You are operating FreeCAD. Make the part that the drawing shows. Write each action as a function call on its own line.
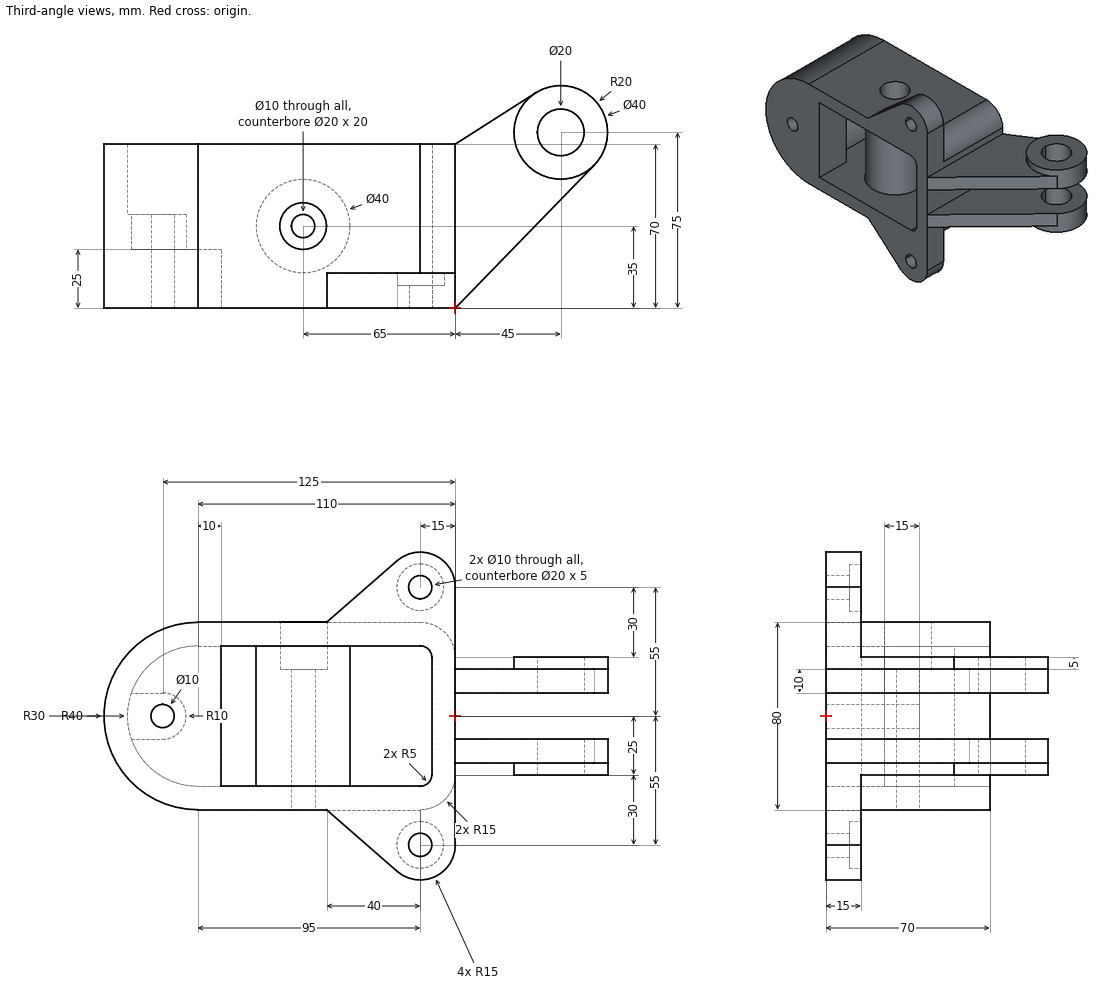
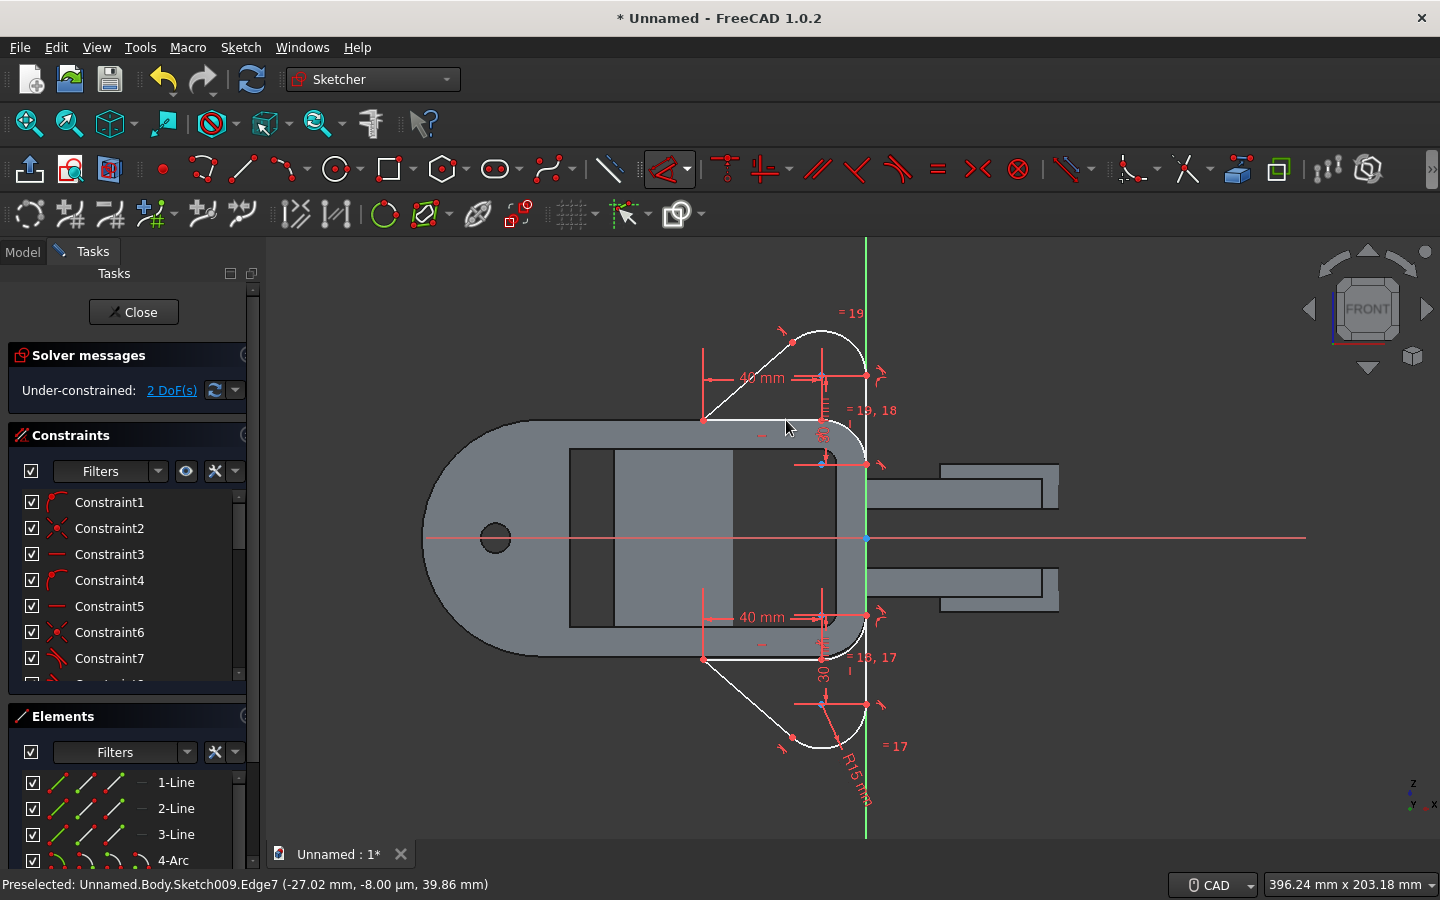
click(866, 615)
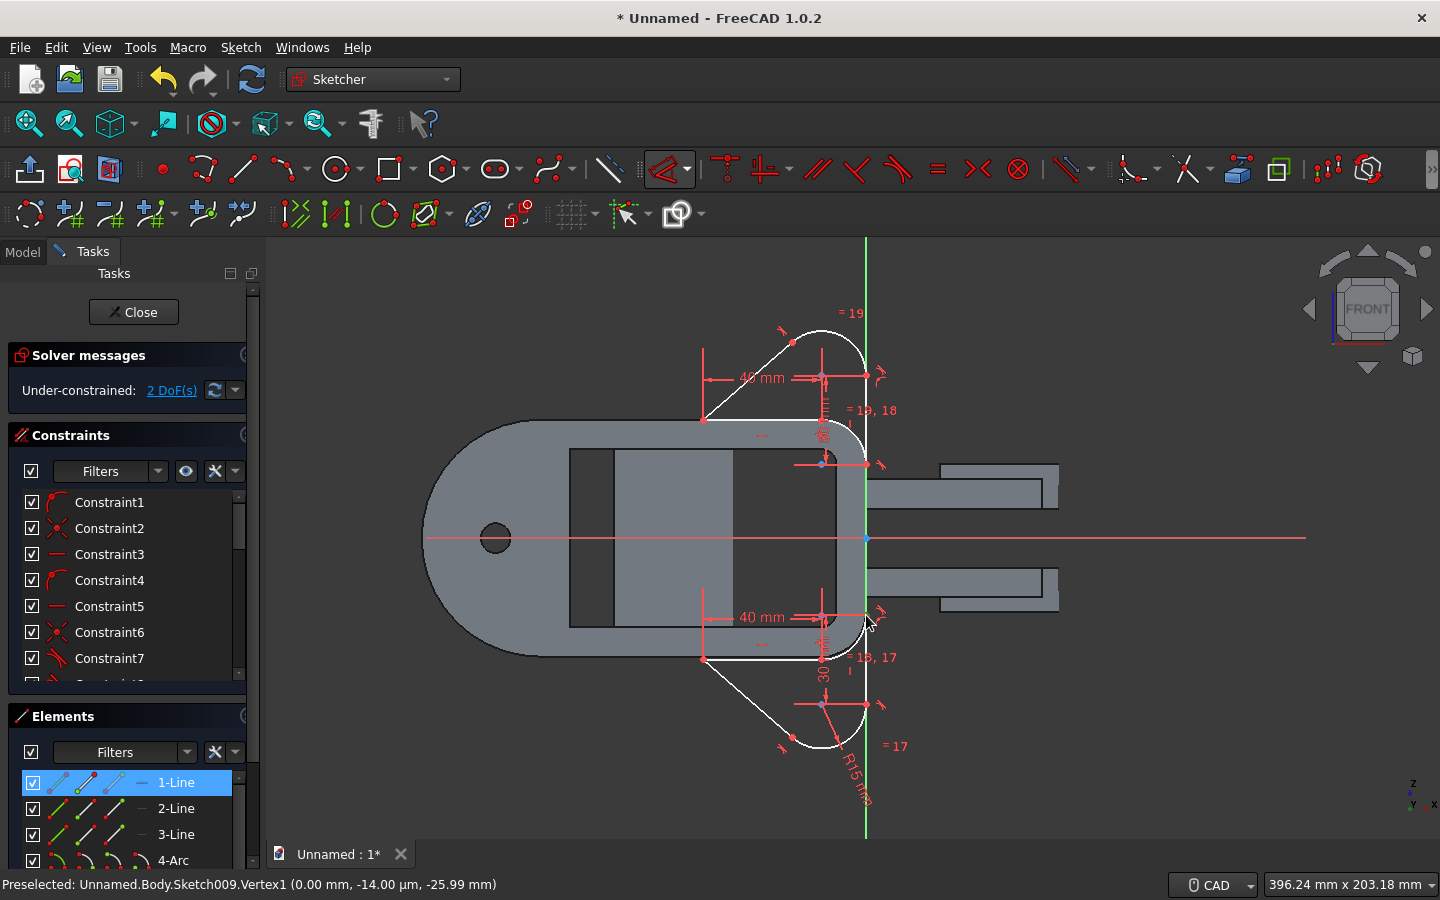
key(i)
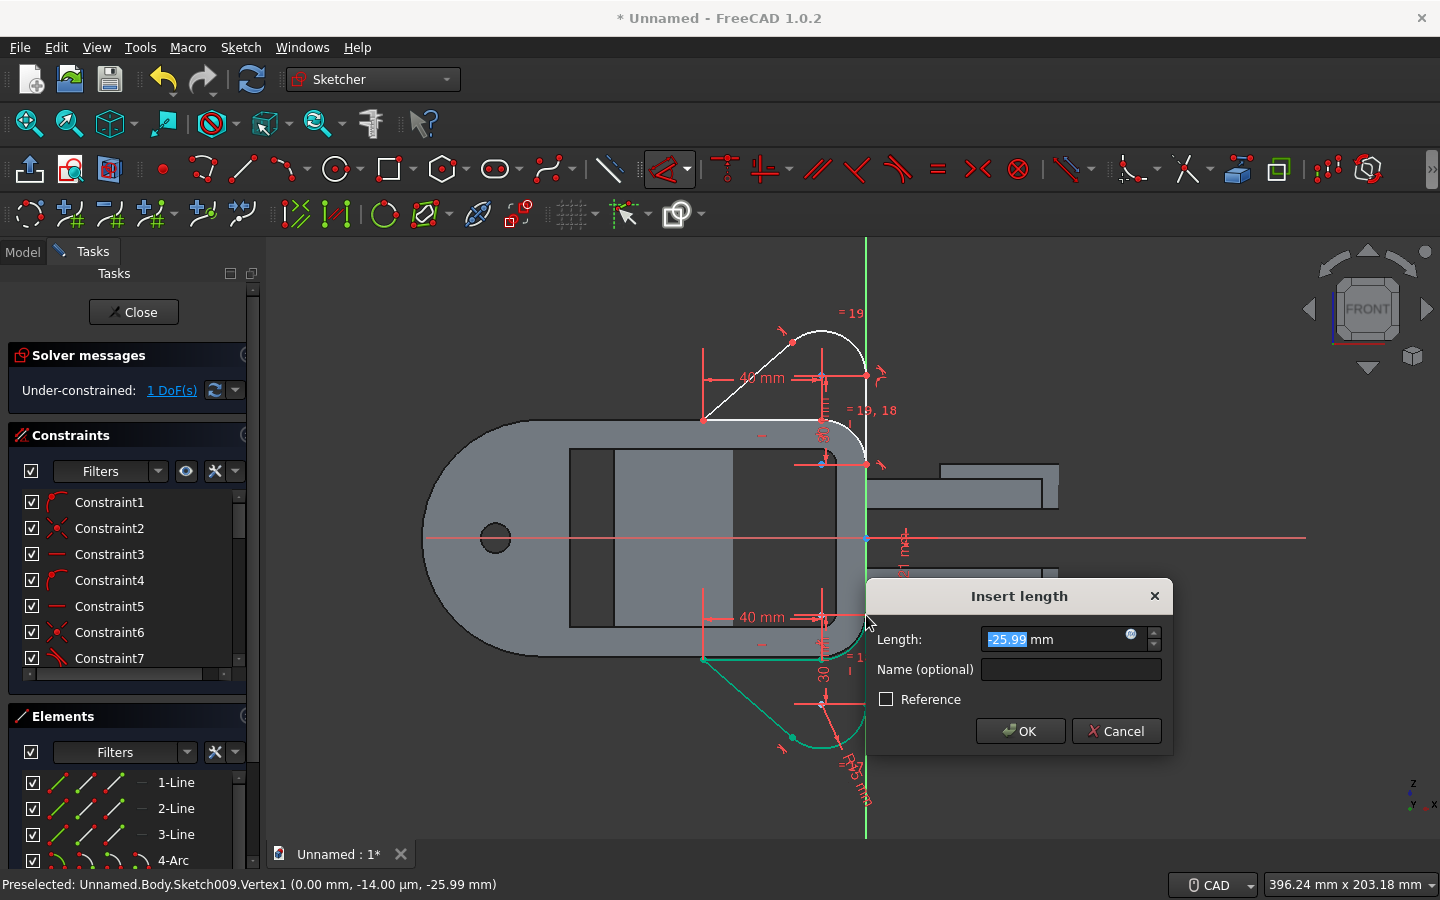
text(-25)
key(Return)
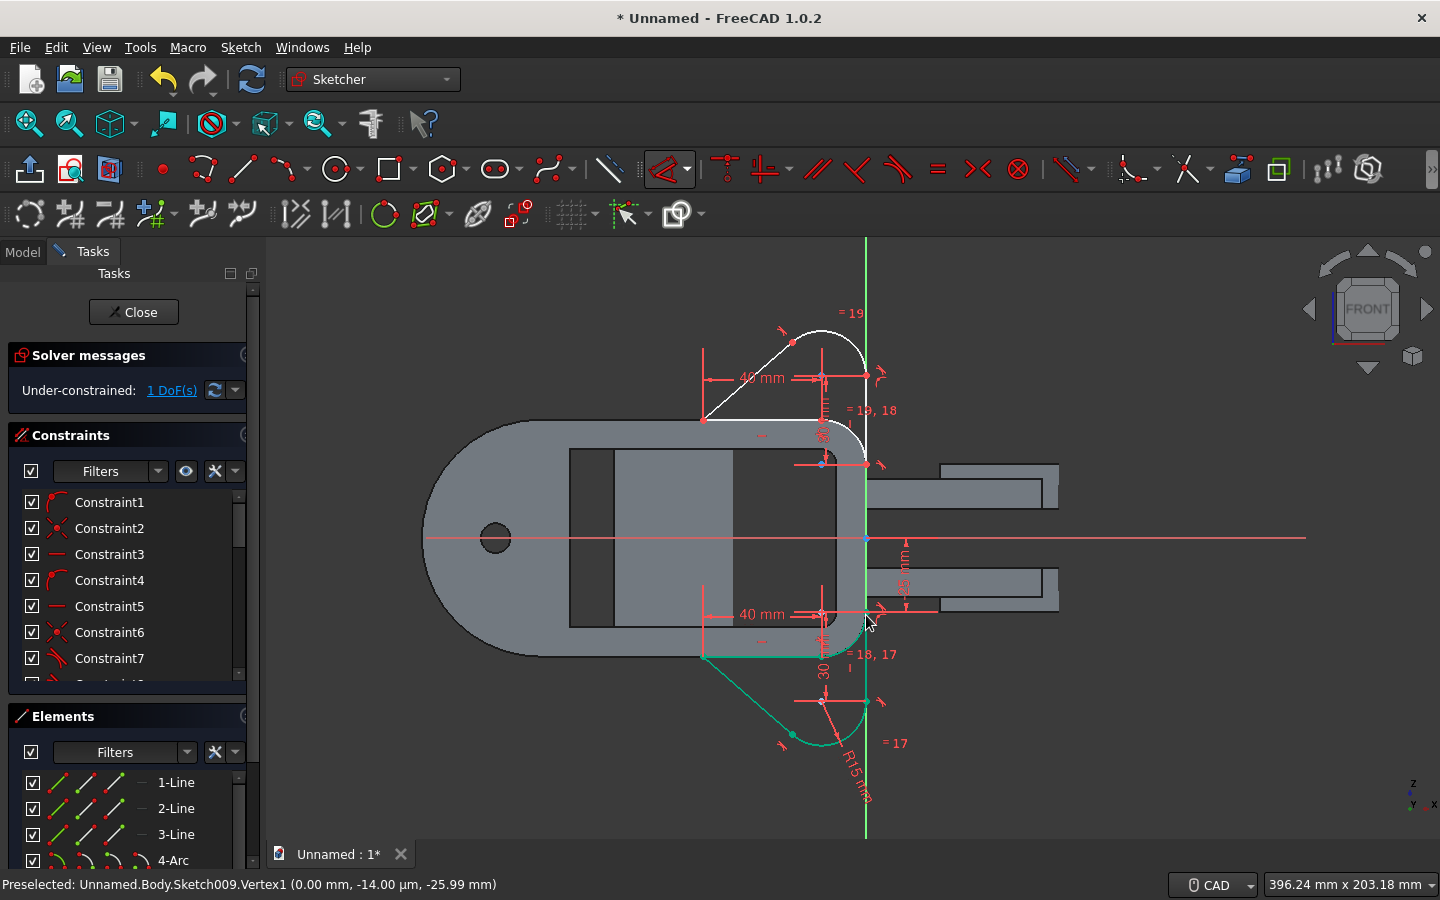
click(866, 376)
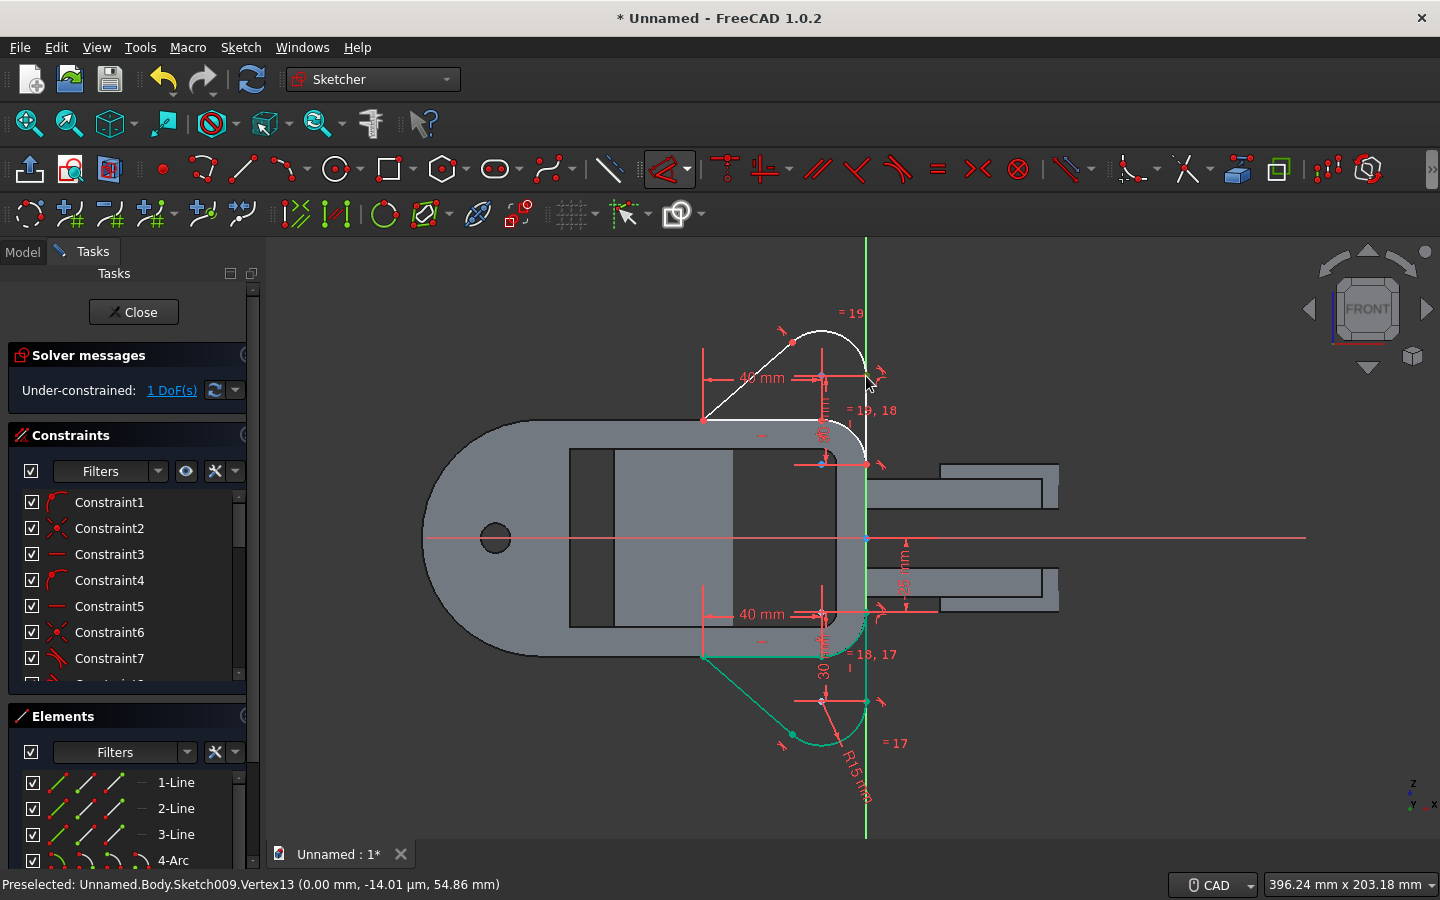
key(i)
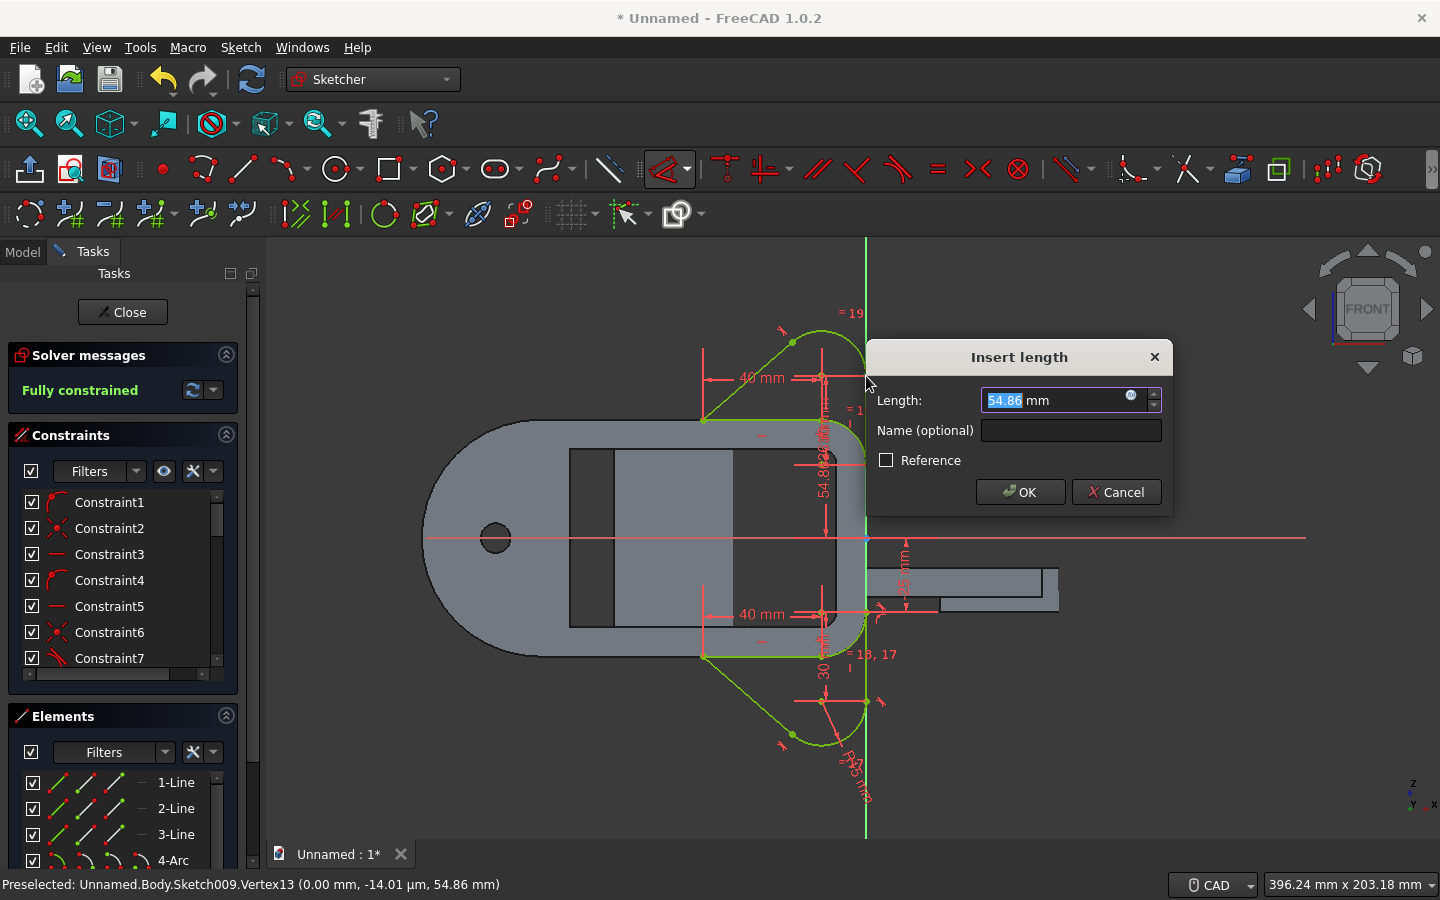
text(55)
key(Return)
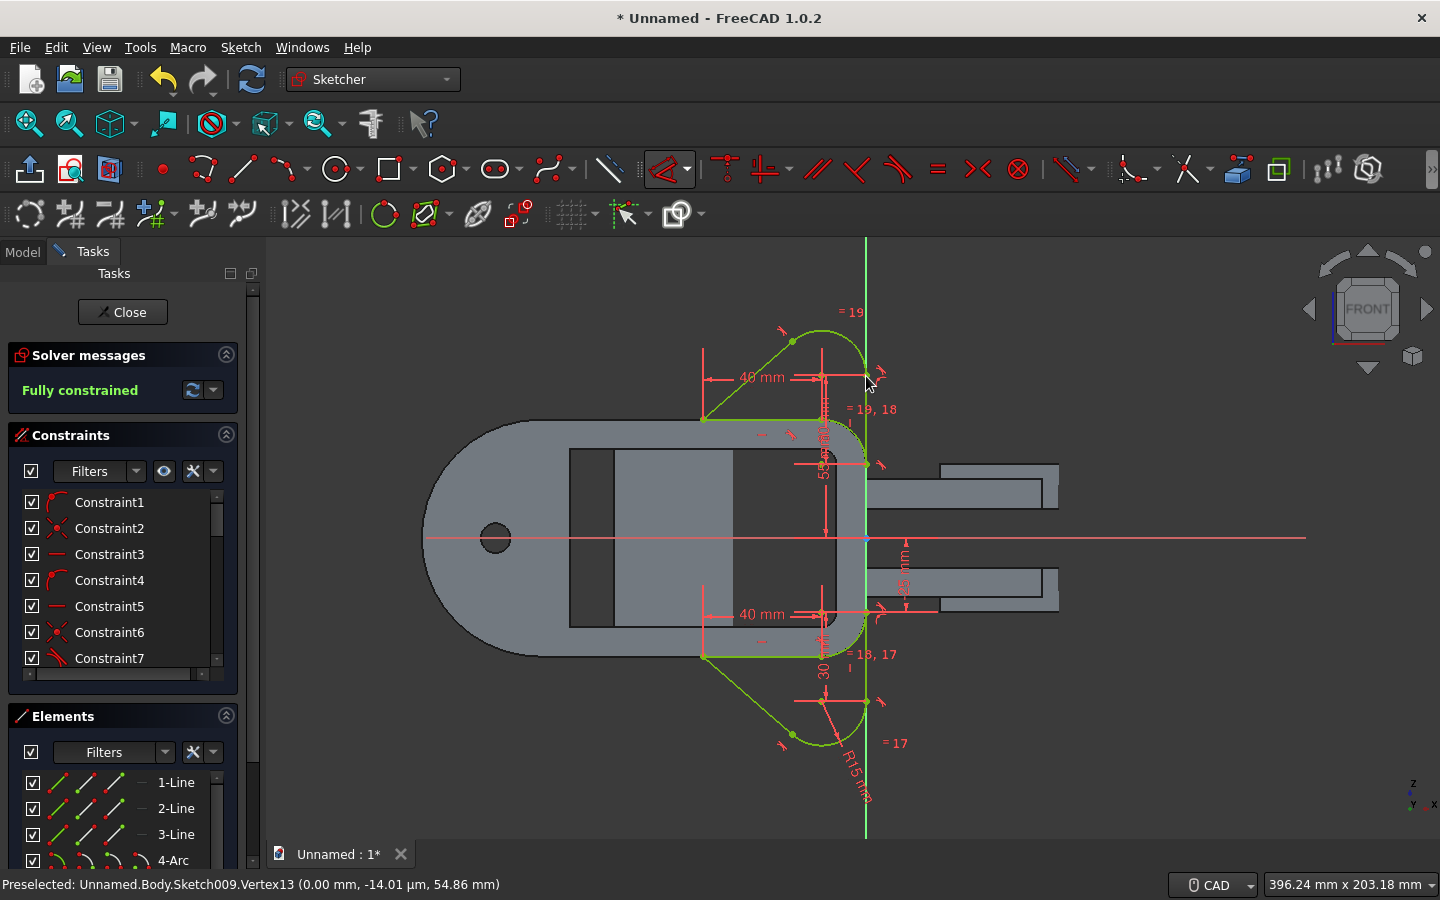
click(123, 312)